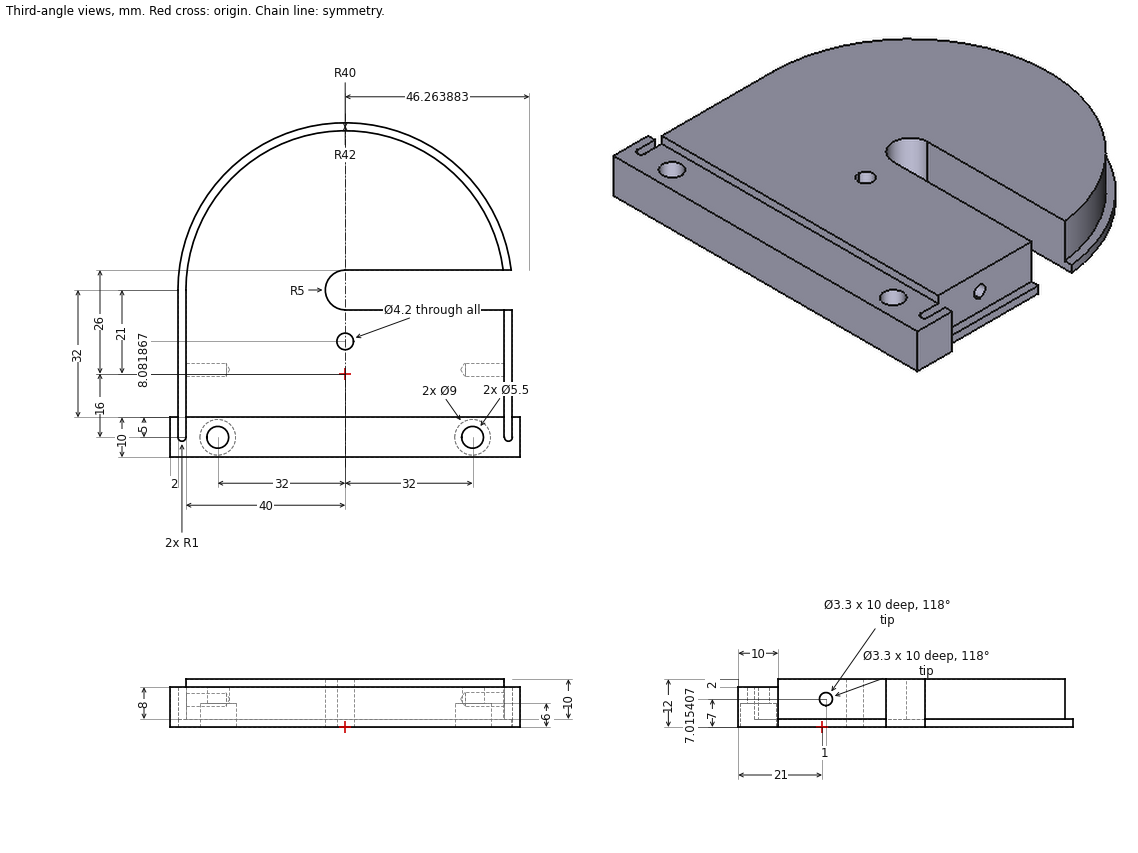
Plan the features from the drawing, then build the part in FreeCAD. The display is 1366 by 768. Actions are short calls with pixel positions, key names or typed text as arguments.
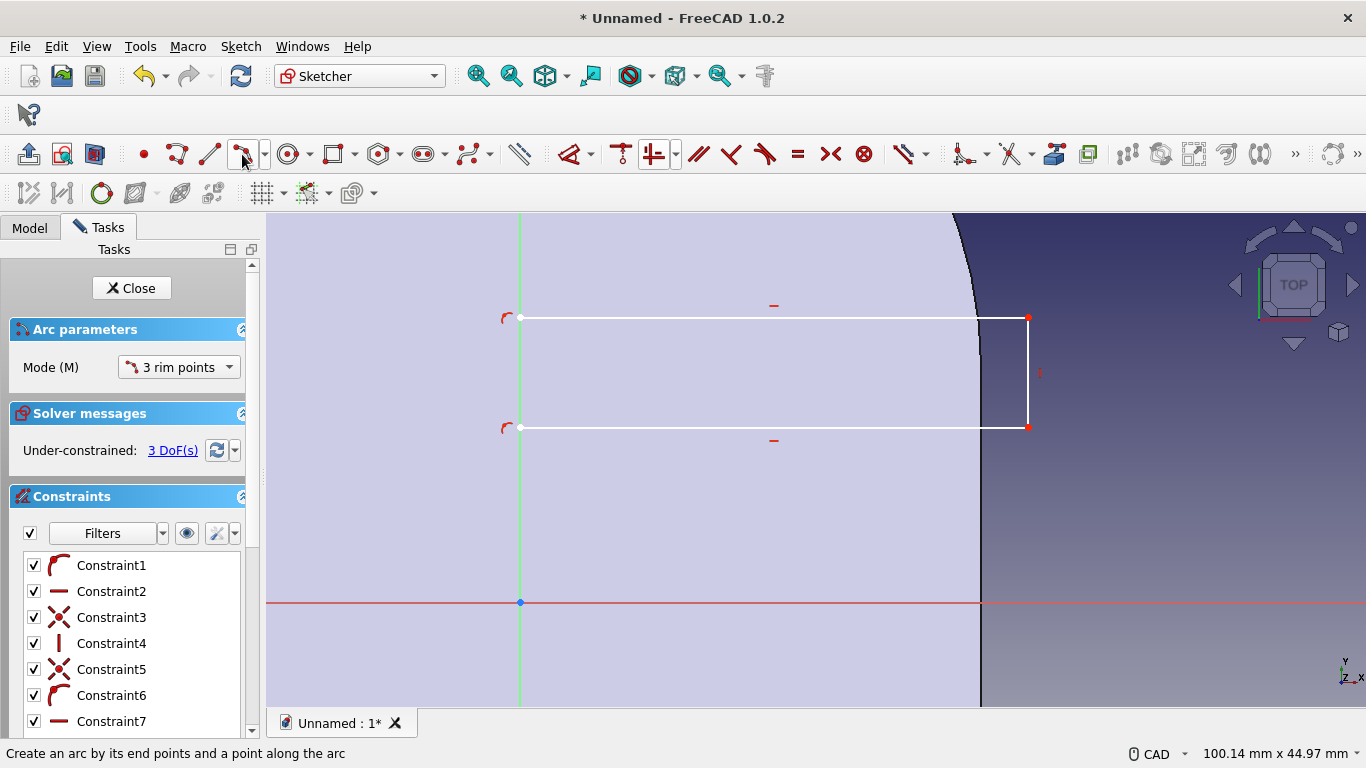
click(520, 428)
click(520, 318)
click(465, 372)
key(Escape)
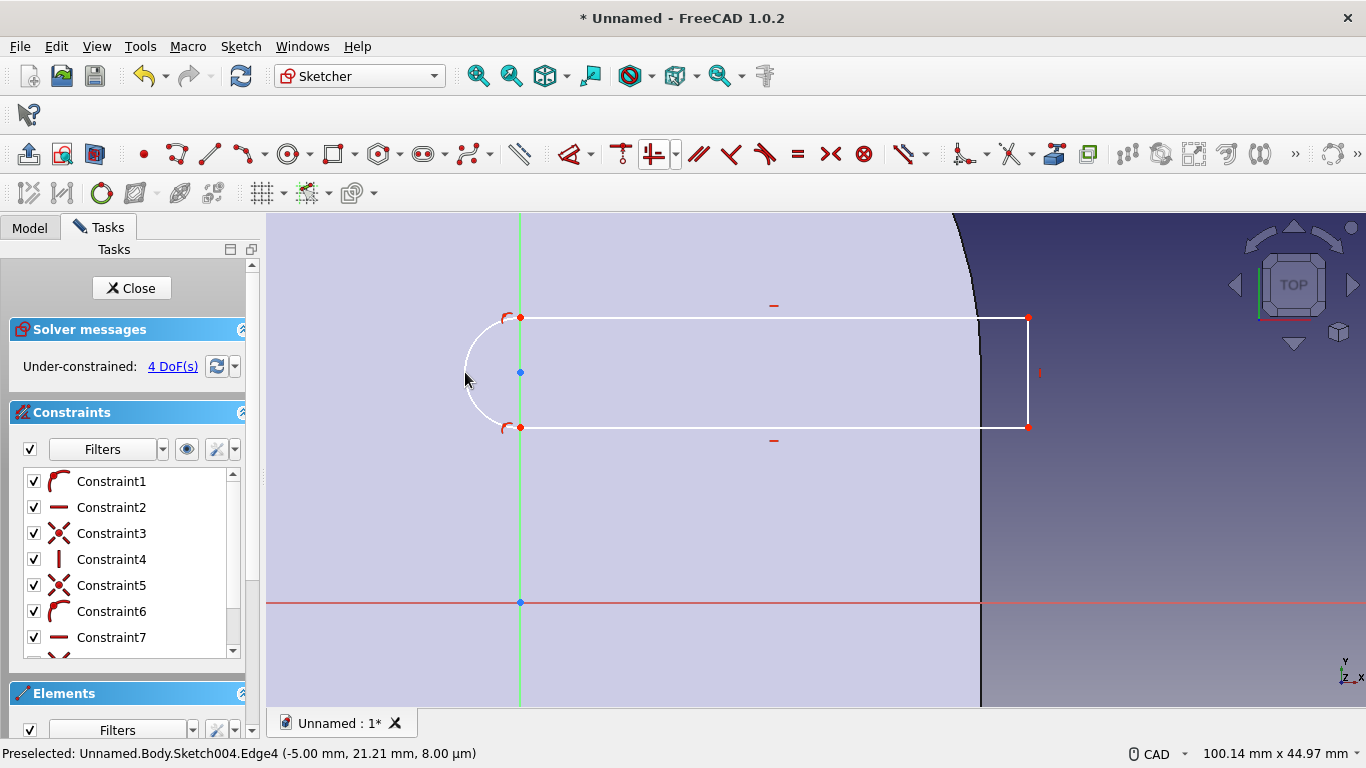
click(672, 318)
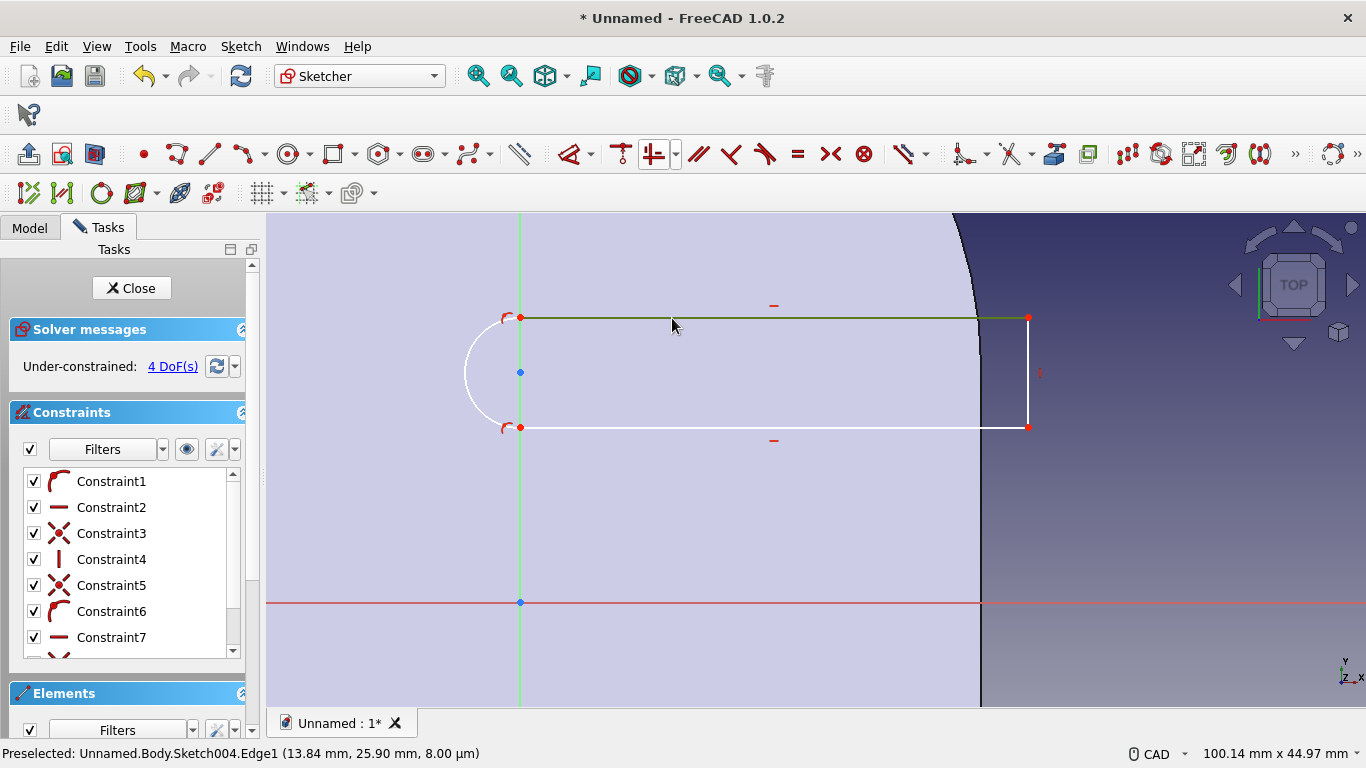
click(476, 341)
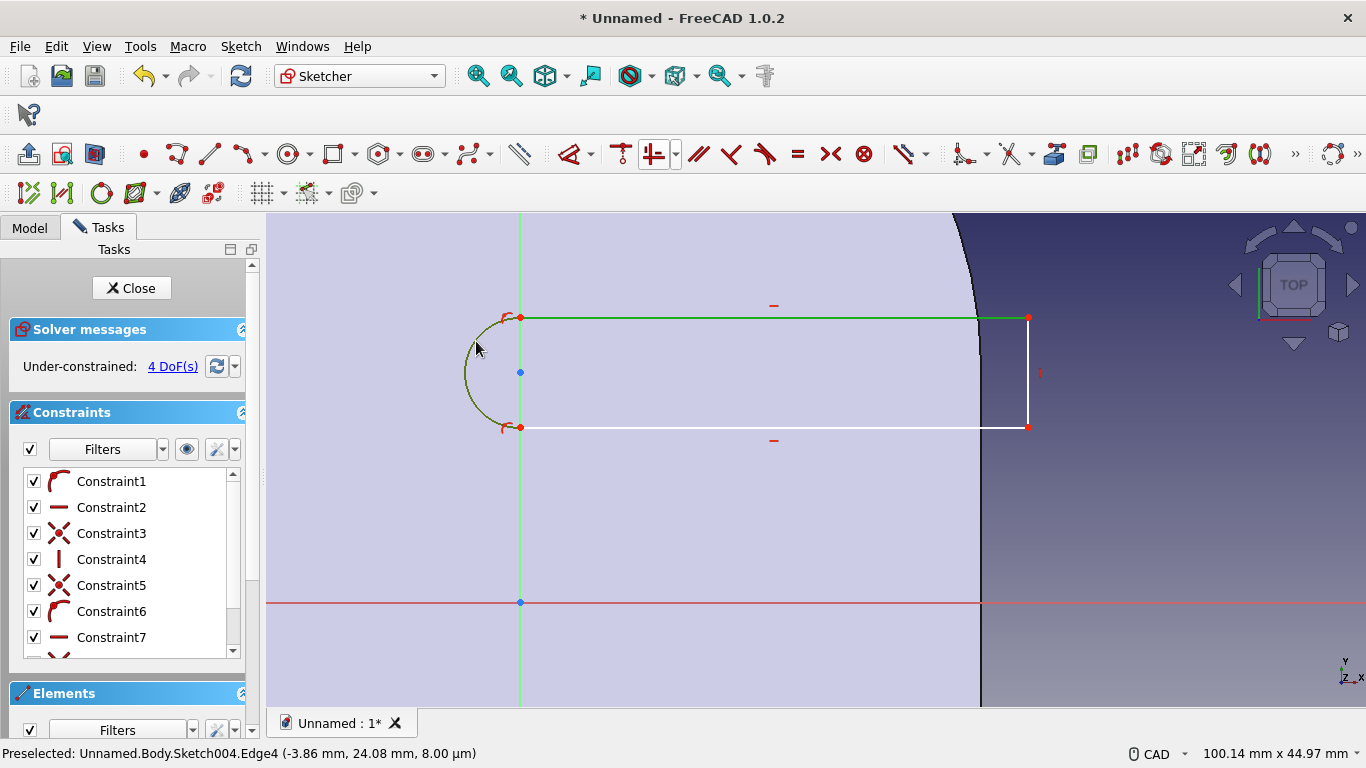
click(765, 154)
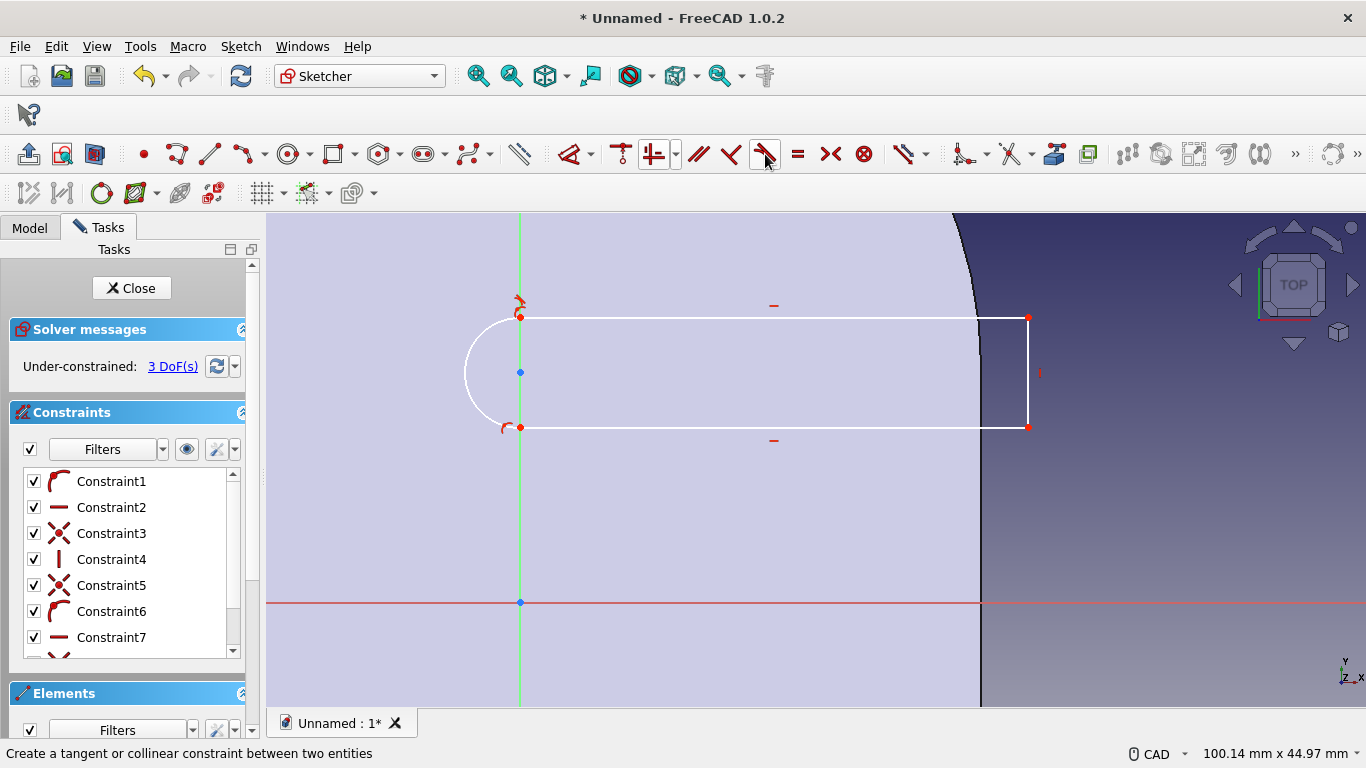
click(568, 154)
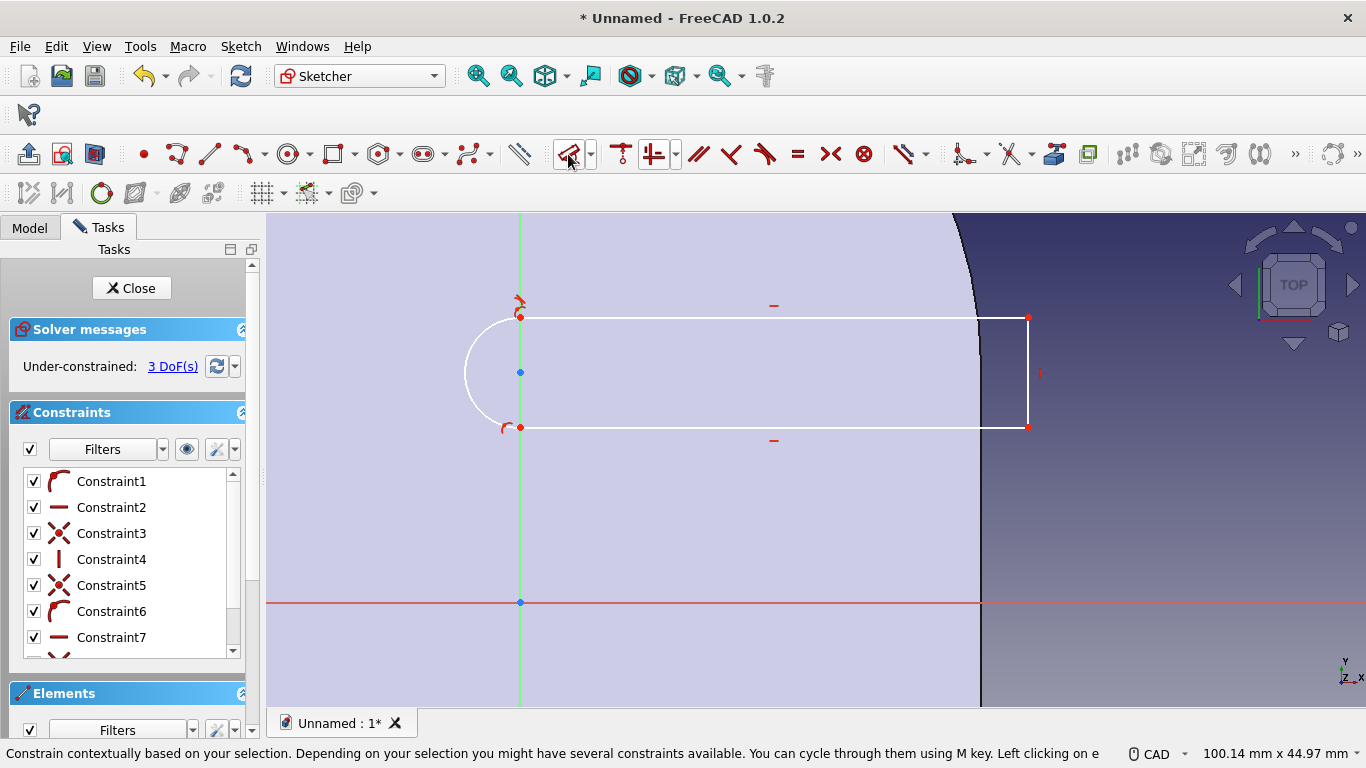
click(476, 341)
click(450, 322)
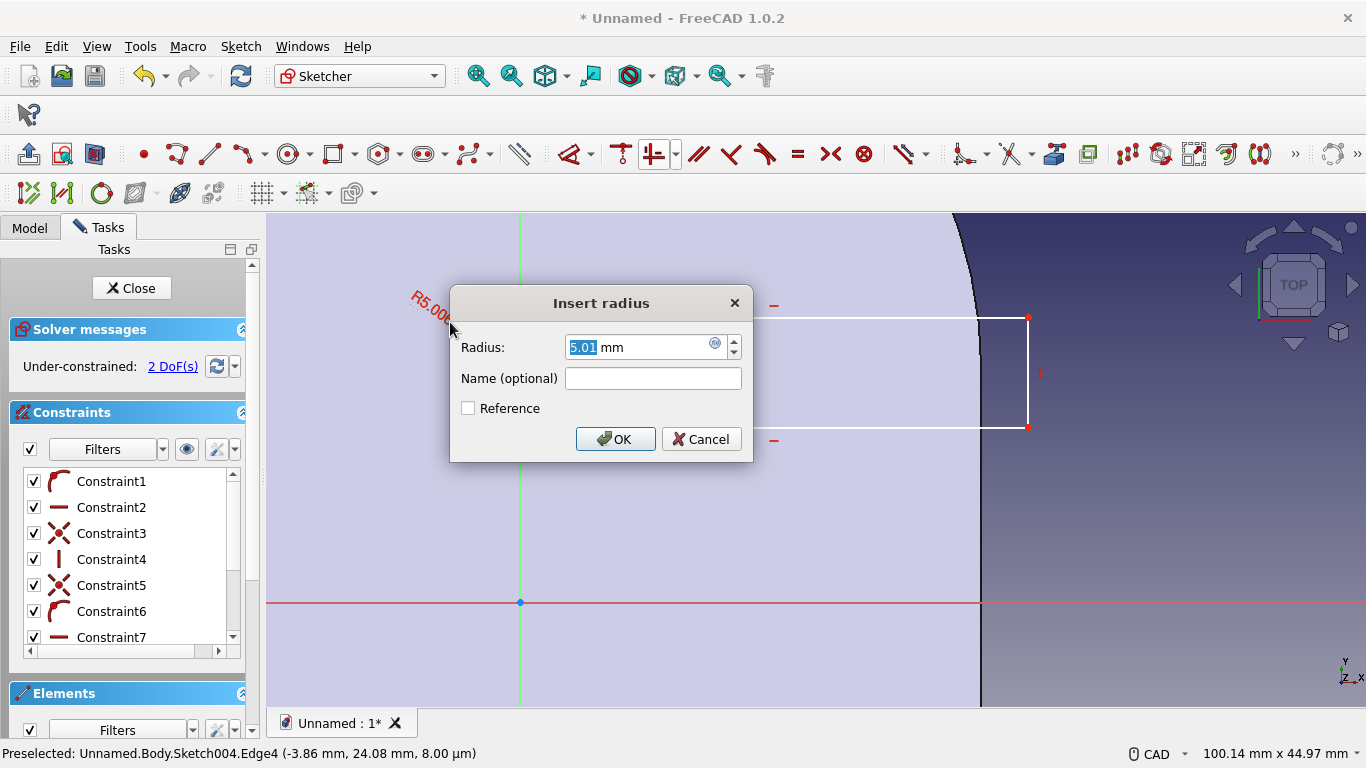
text(5)
key(Return)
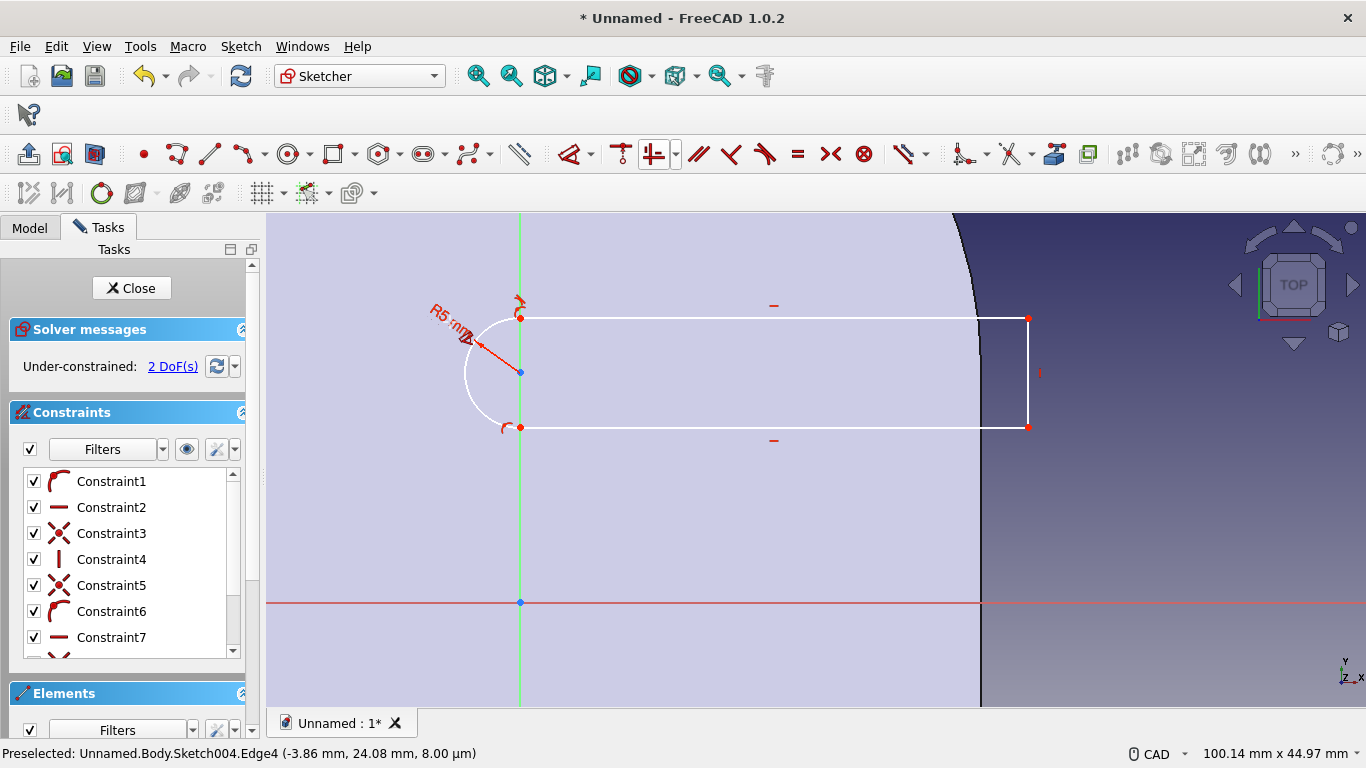
click(520, 318)
click(486, 460)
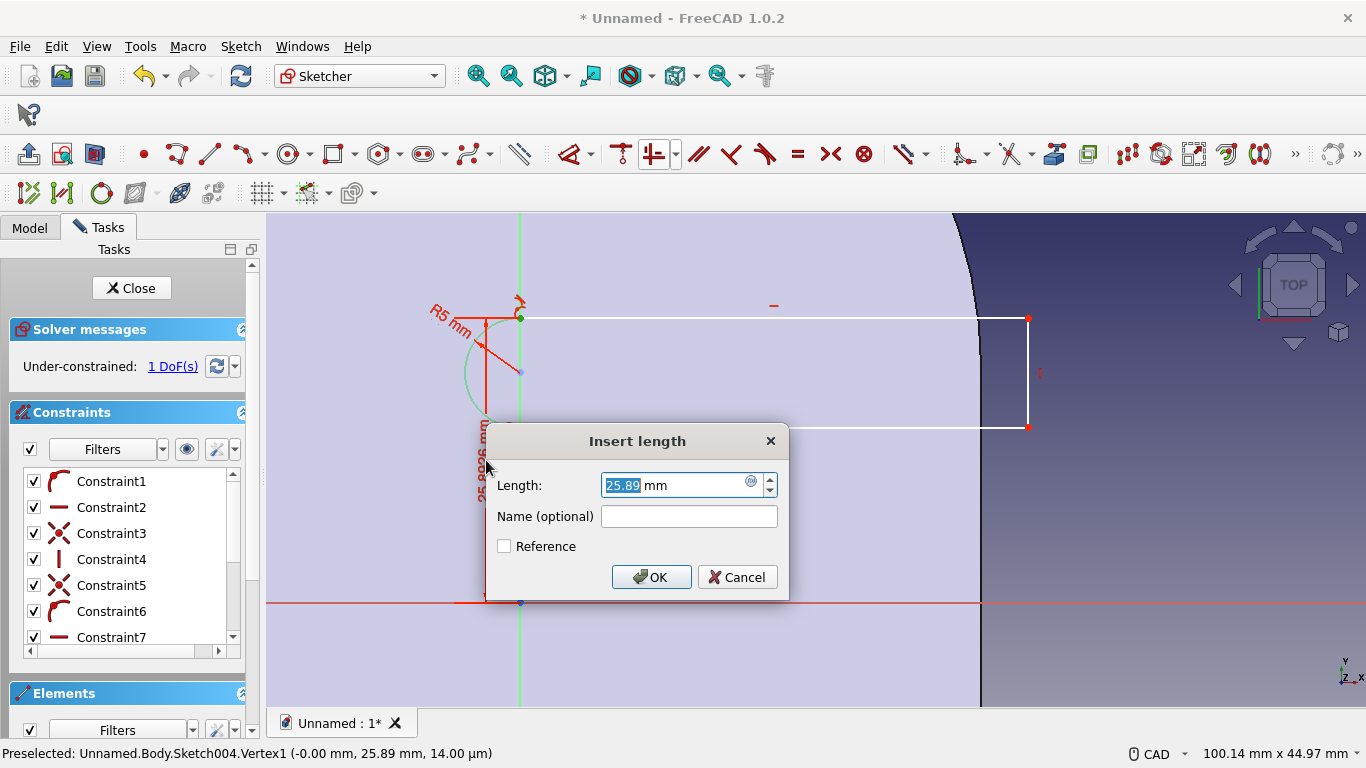
text(26)
key(Return)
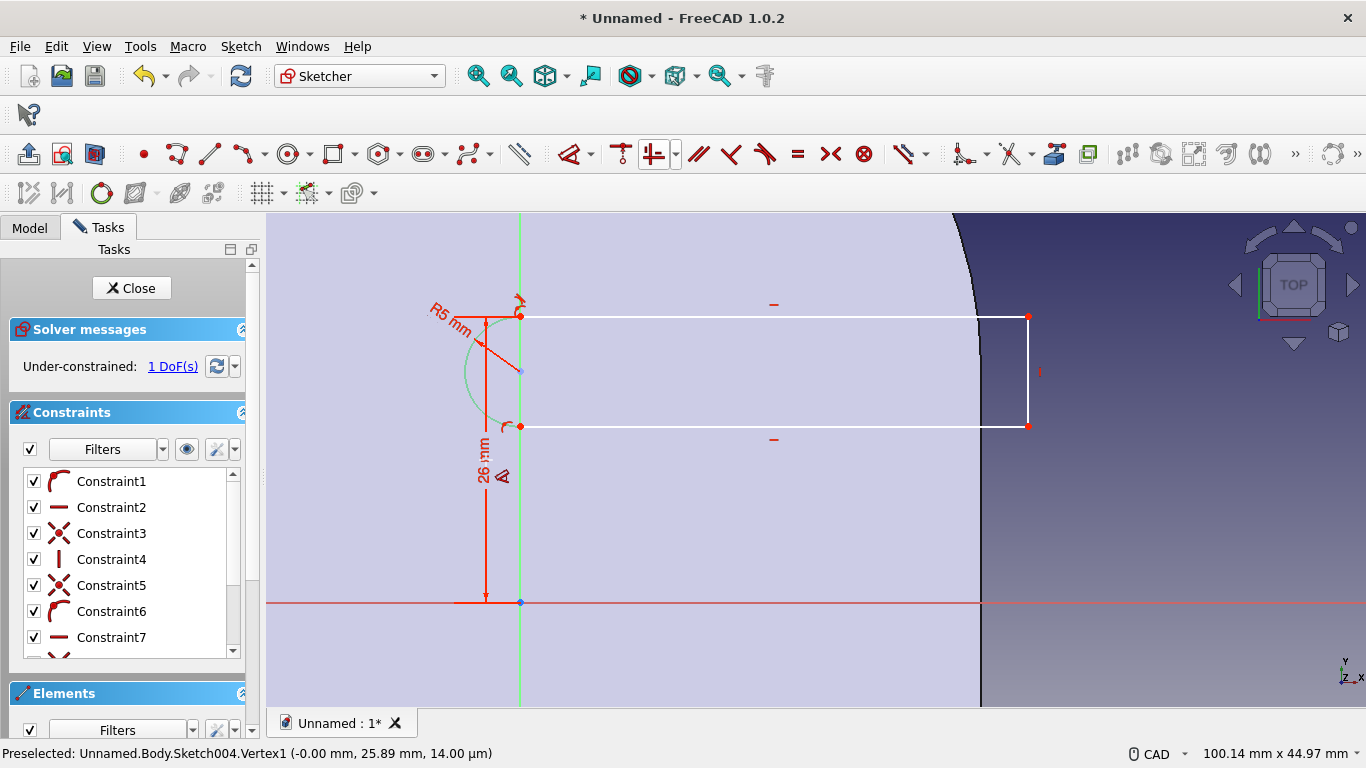
click(672, 317)
click(774, 283)